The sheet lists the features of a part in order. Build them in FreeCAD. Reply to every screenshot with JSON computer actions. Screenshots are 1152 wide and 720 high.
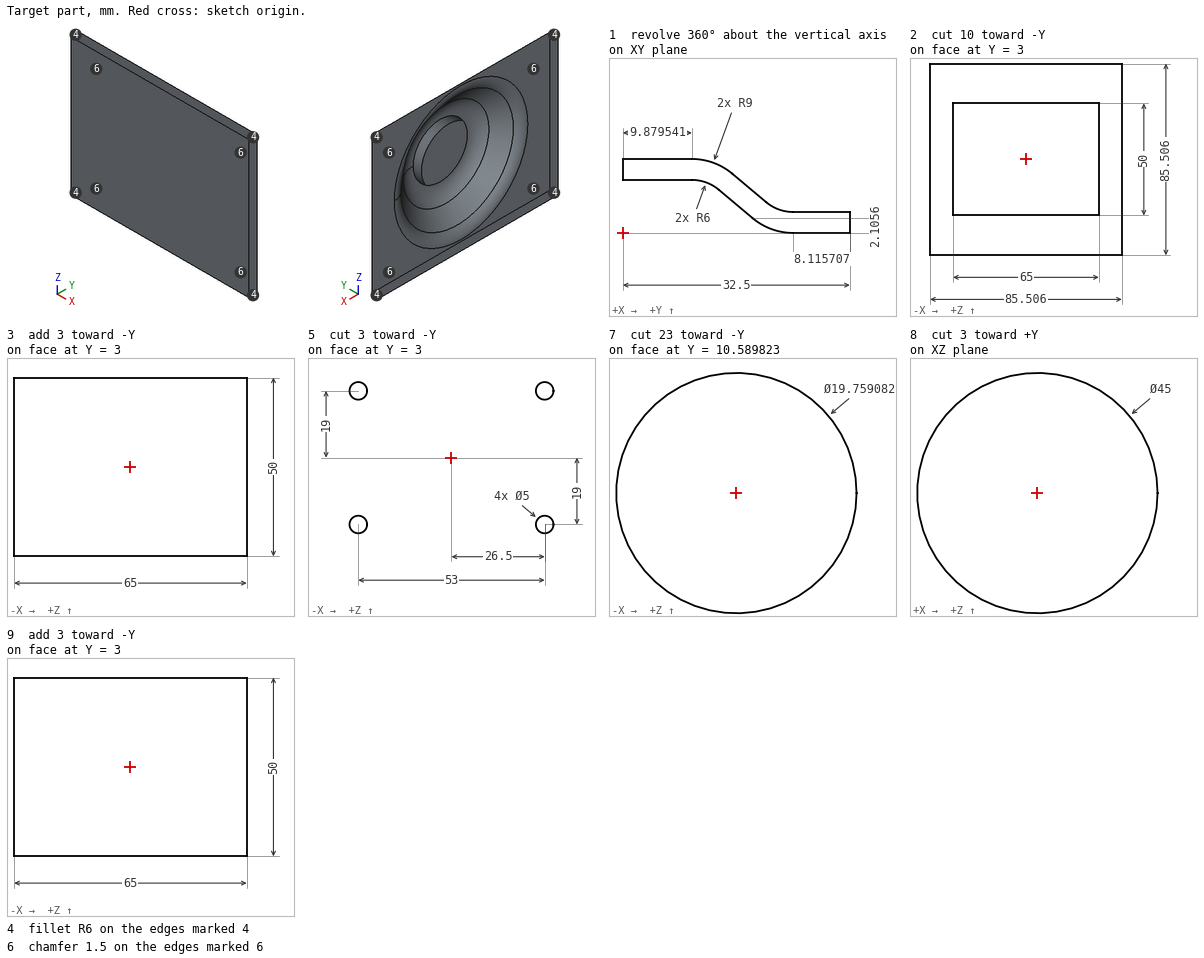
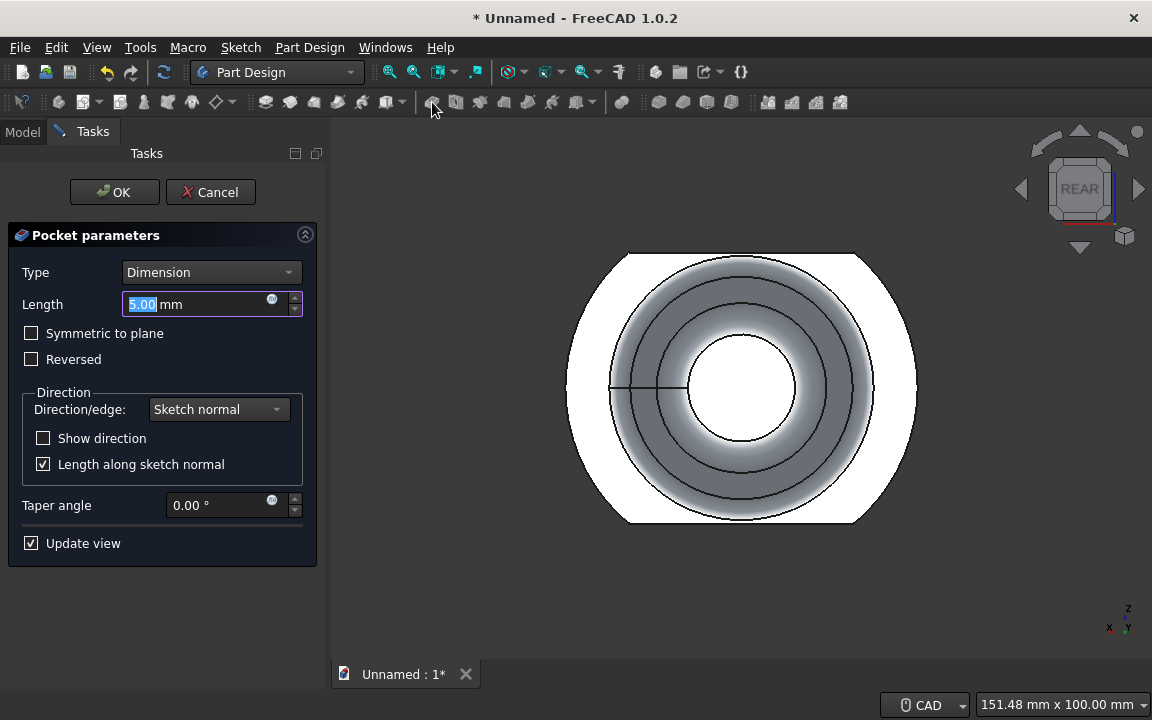
{"action": "type", "text": "10"}
{"action": "key", "text": "Tab"}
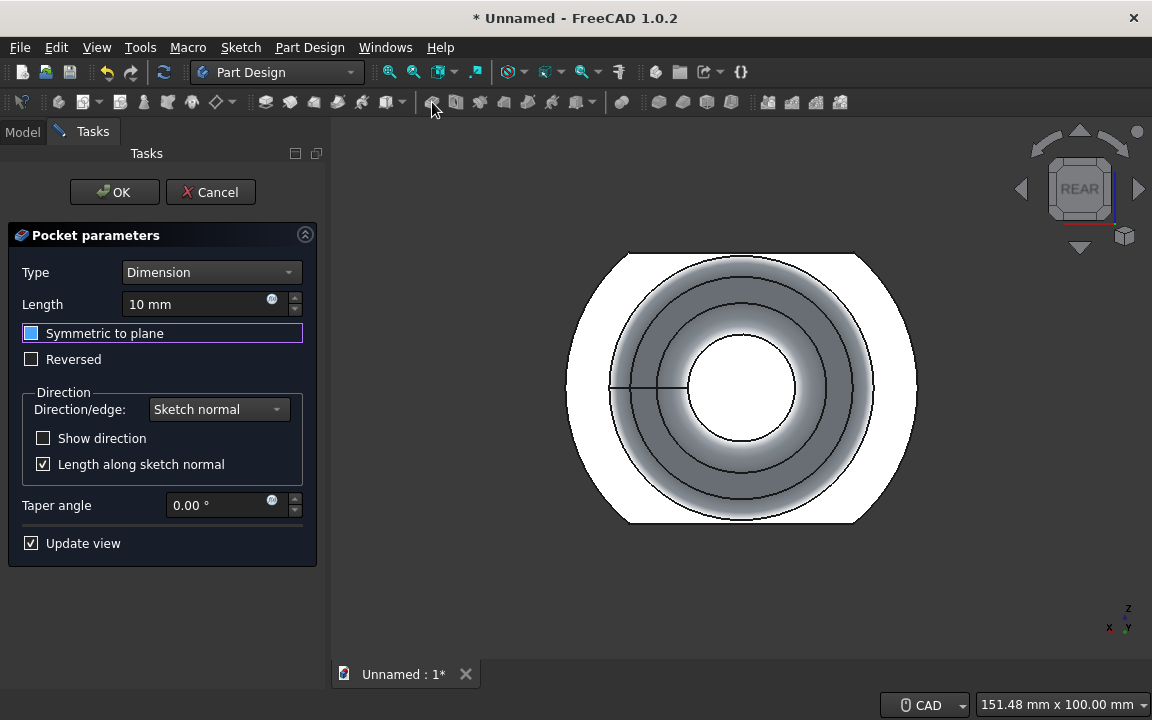
{"action": "left_click", "coordinate": [115, 192]}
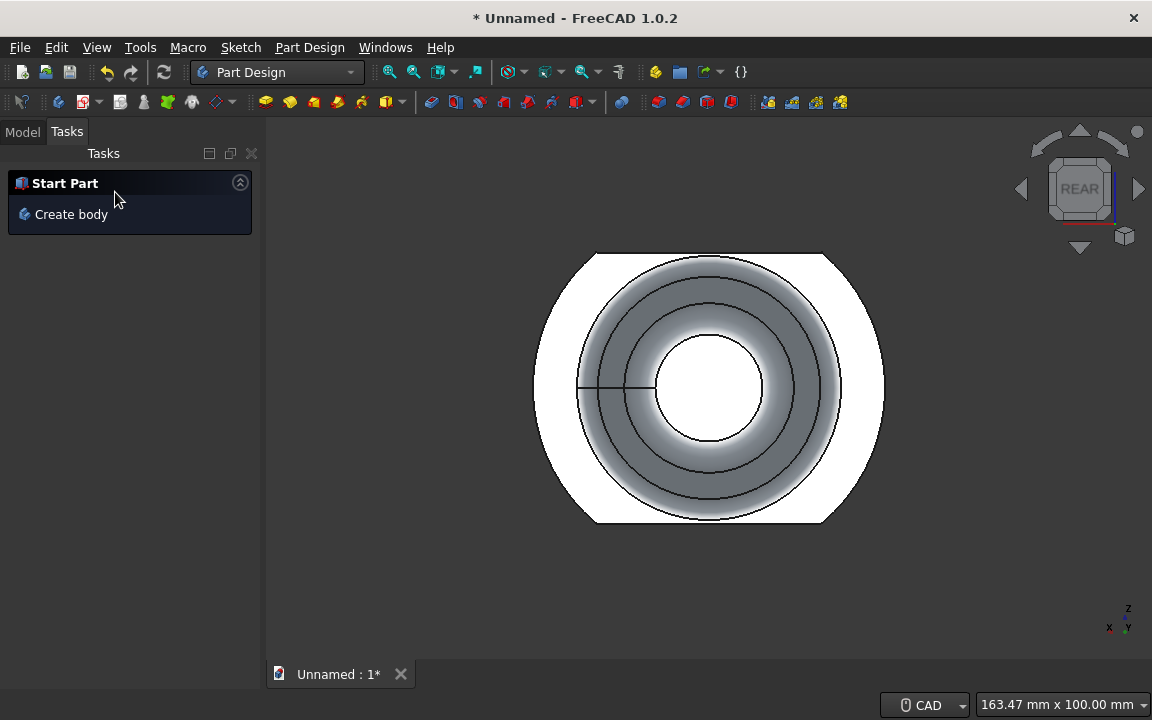
{"action": "left_click", "coordinate": [558, 426]}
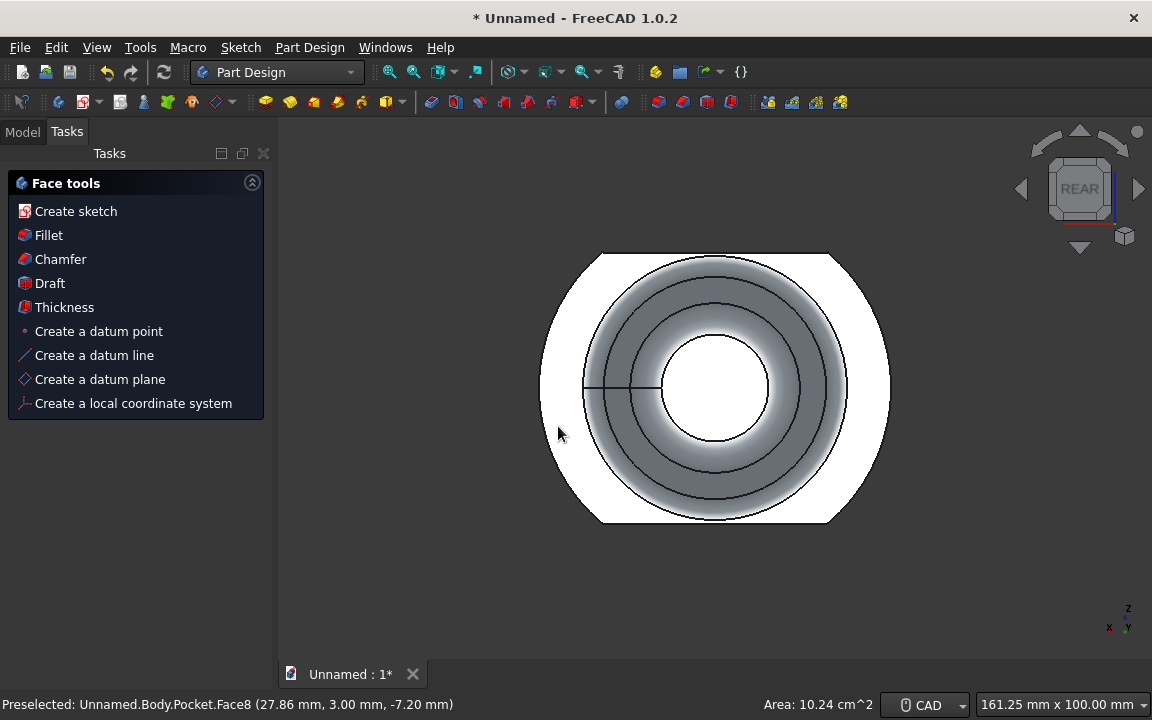
{"action": "left_click", "coordinate": [84, 102]}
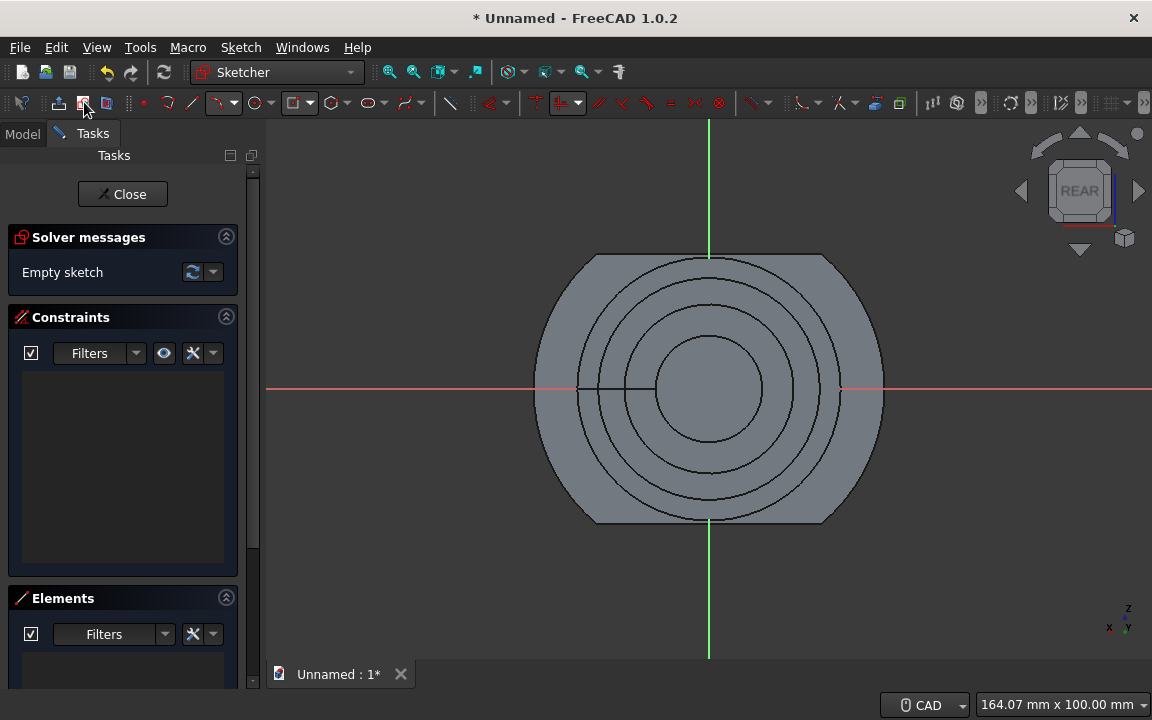
{"action": "left_click", "coordinate": [108, 104]}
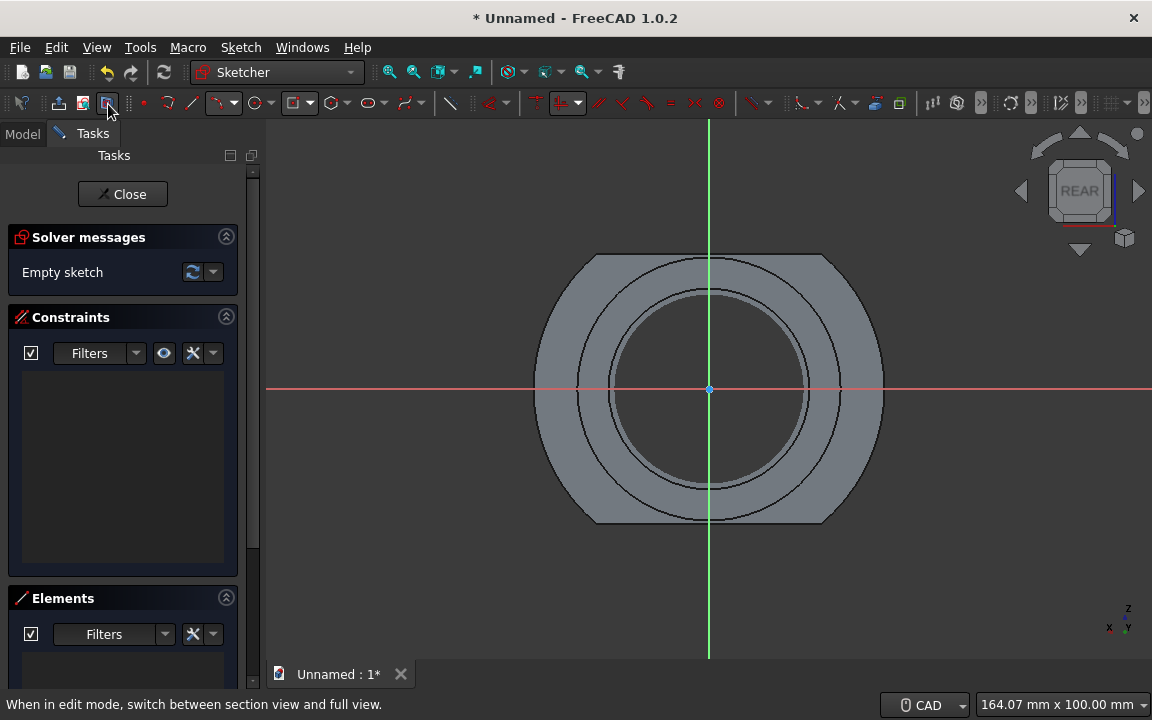
{"action": "left_click", "coordinate": [294, 104]}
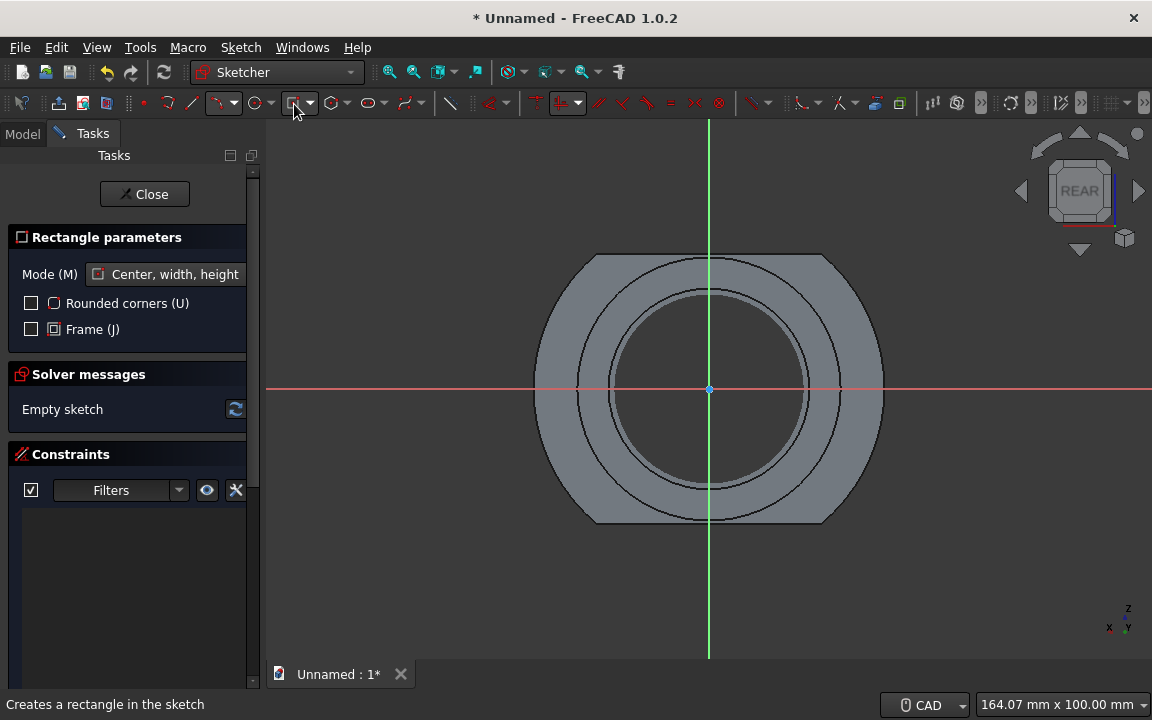
{"action": "left_click", "coordinate": [709, 389]}
{"action": "left_click", "coordinate": [885, 254]}
{"action": "key", "text": "Escape"}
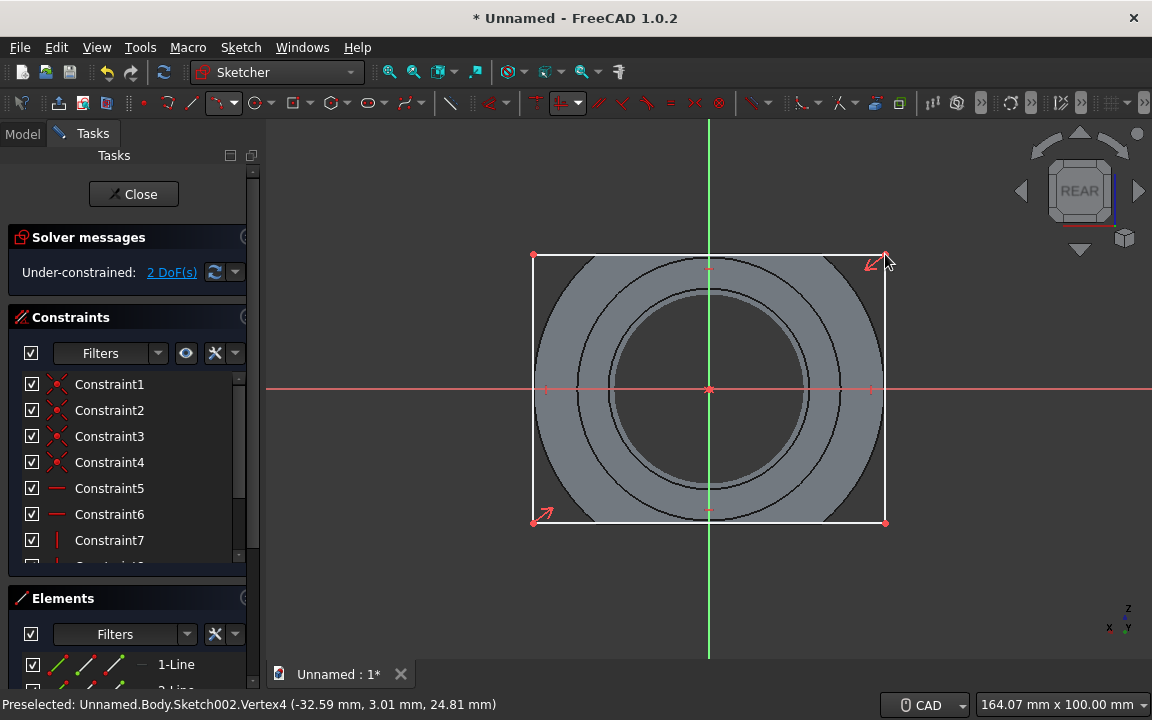
{"action": "left_click", "coordinate": [490, 104]}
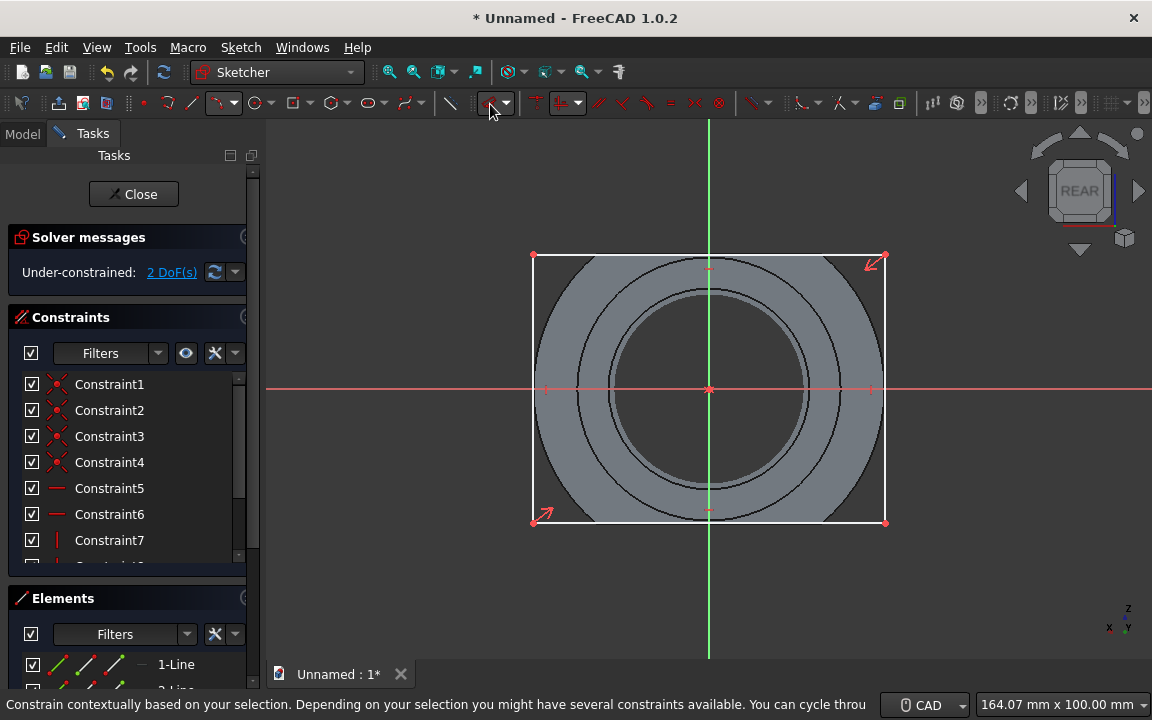
{"action": "left_click", "coordinate": [639, 523]}
{"action": "left_click", "coordinate": [628, 557]}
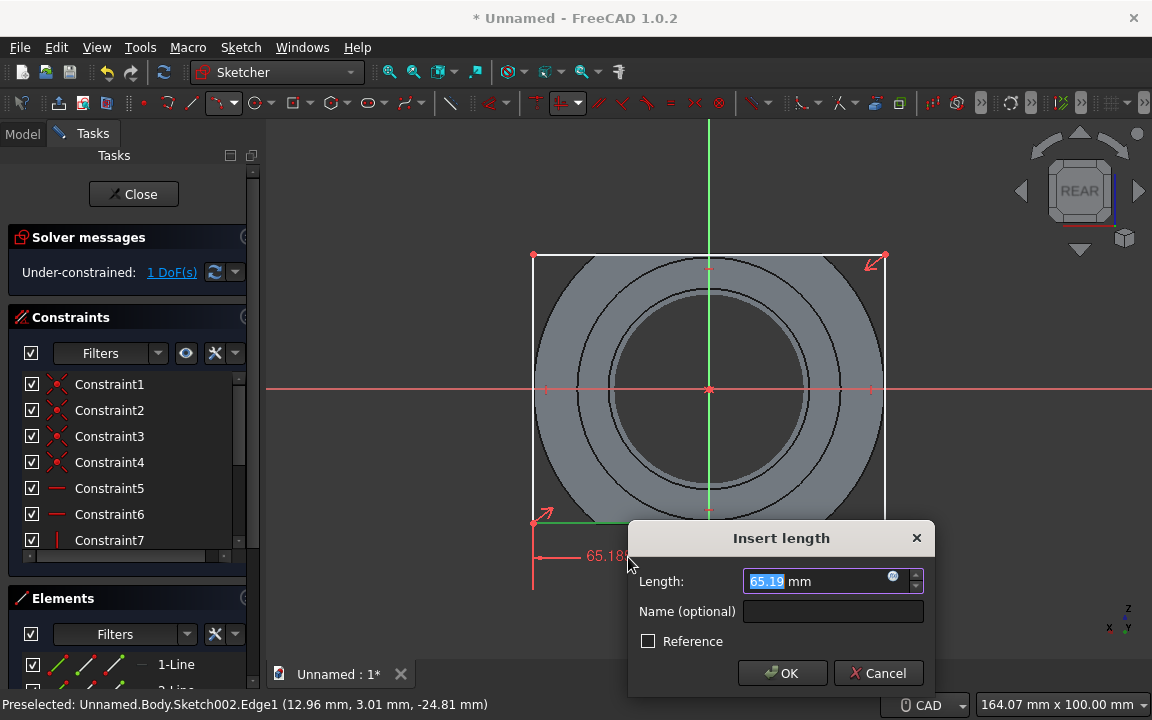
{"action": "type", "text": "65"}
{"action": "key", "text": "Return"}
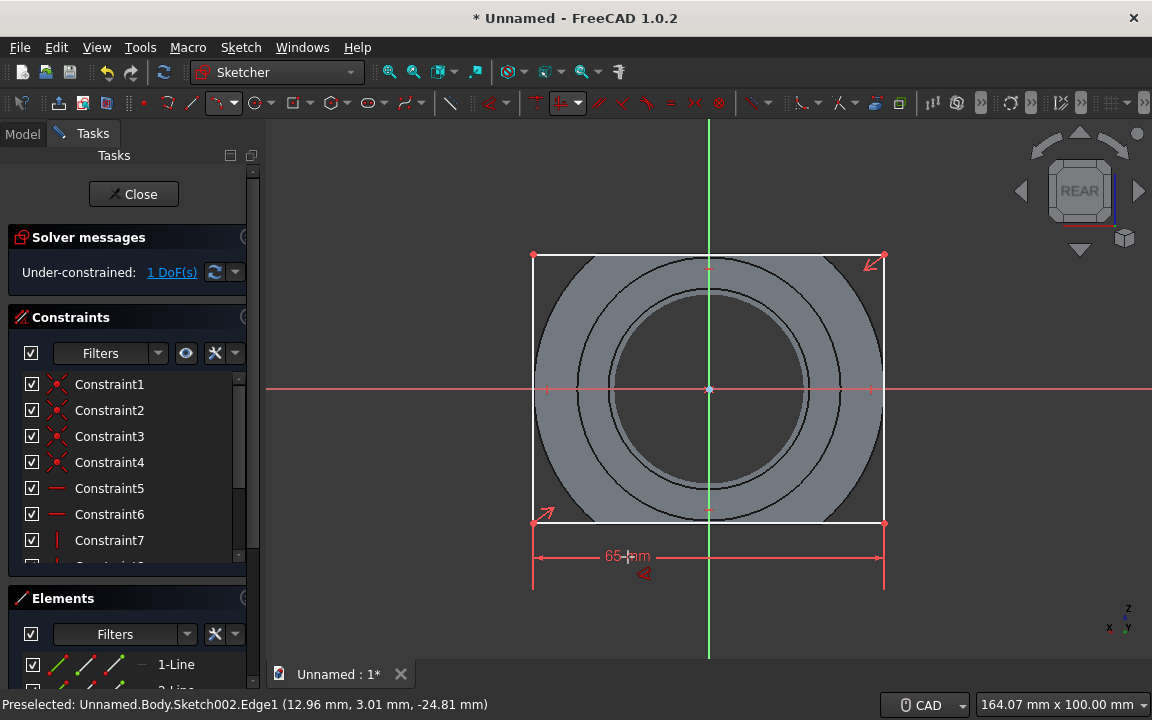
{"action": "left_click", "coordinate": [885, 443]}
{"action": "left_click", "coordinate": [919, 327]}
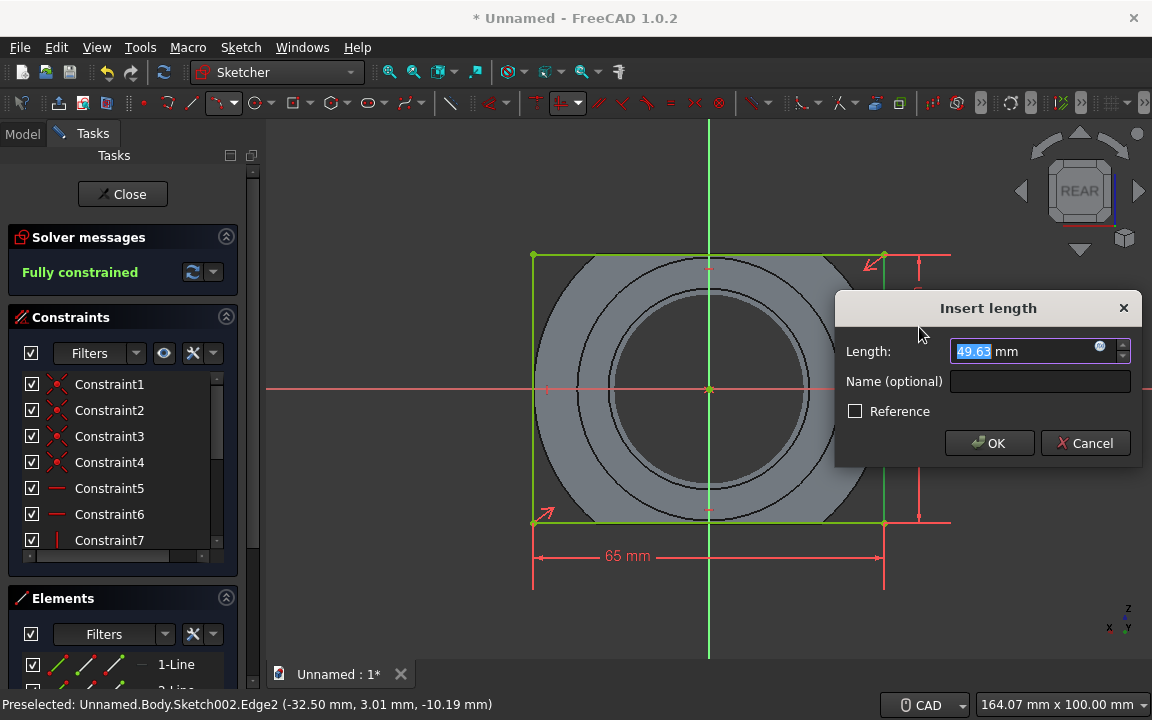
{"action": "type", "text": "50"}
{"action": "key", "text": "Return"}
{"action": "key", "text": "Escape"}